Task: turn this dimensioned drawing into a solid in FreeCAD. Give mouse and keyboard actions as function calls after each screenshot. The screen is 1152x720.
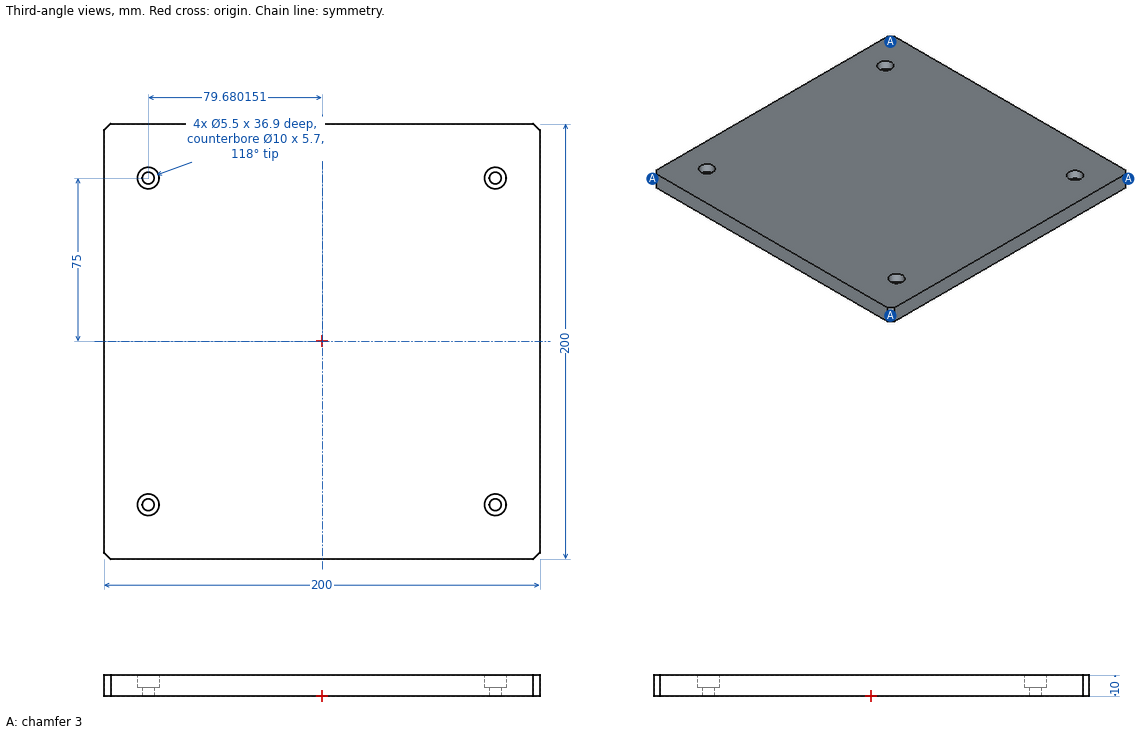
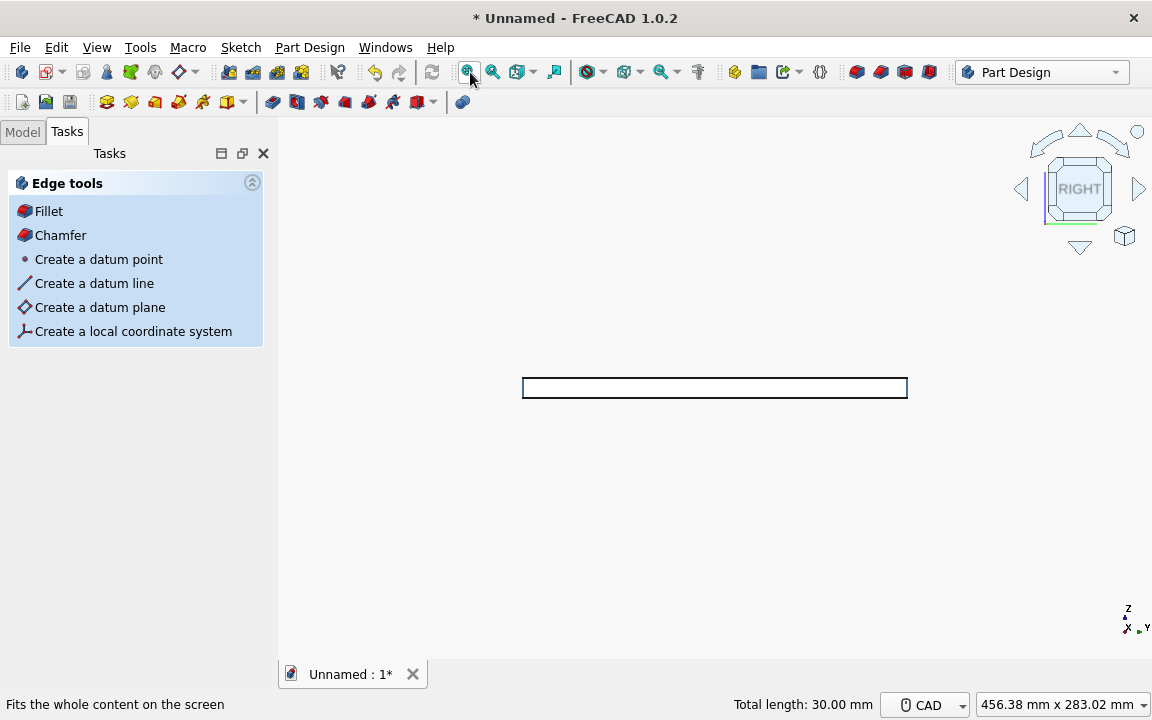
key(5)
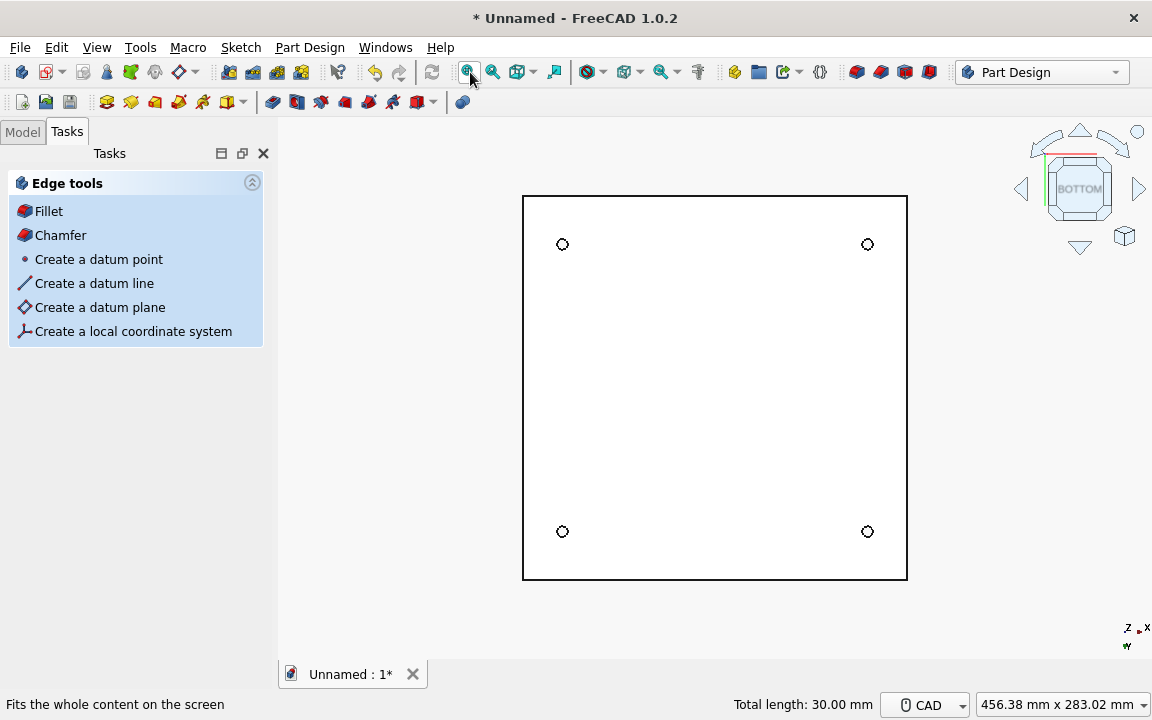
scroll(523, 579, up, 4)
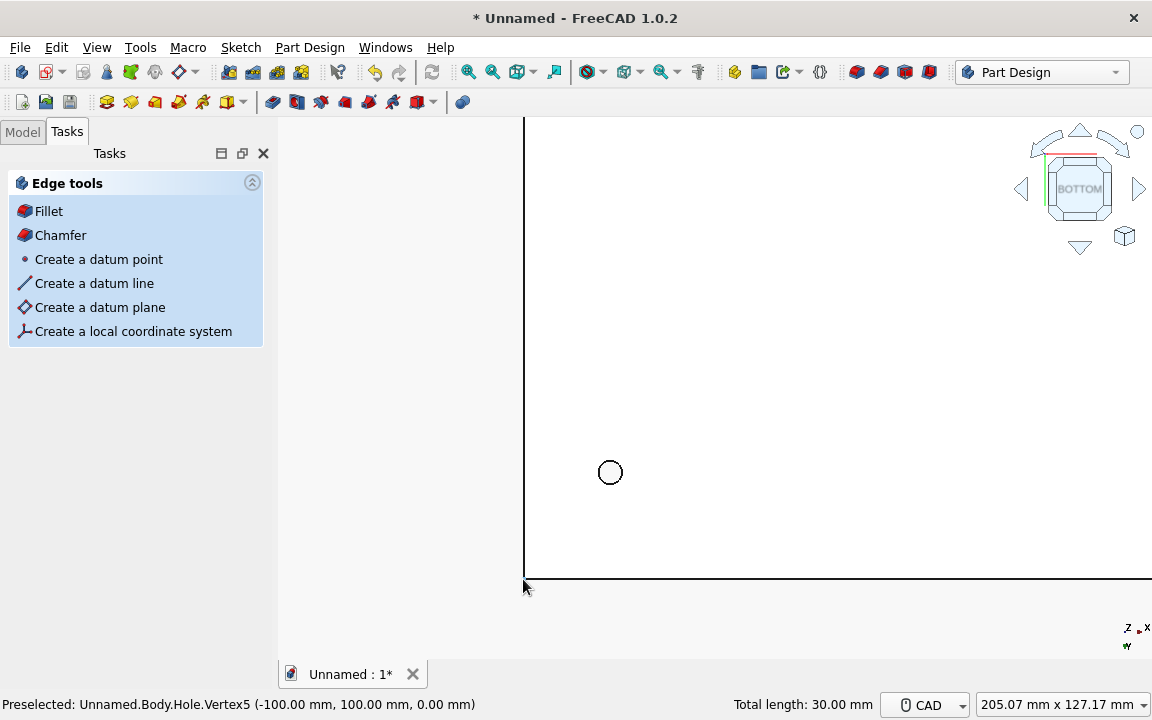
click(470, 72)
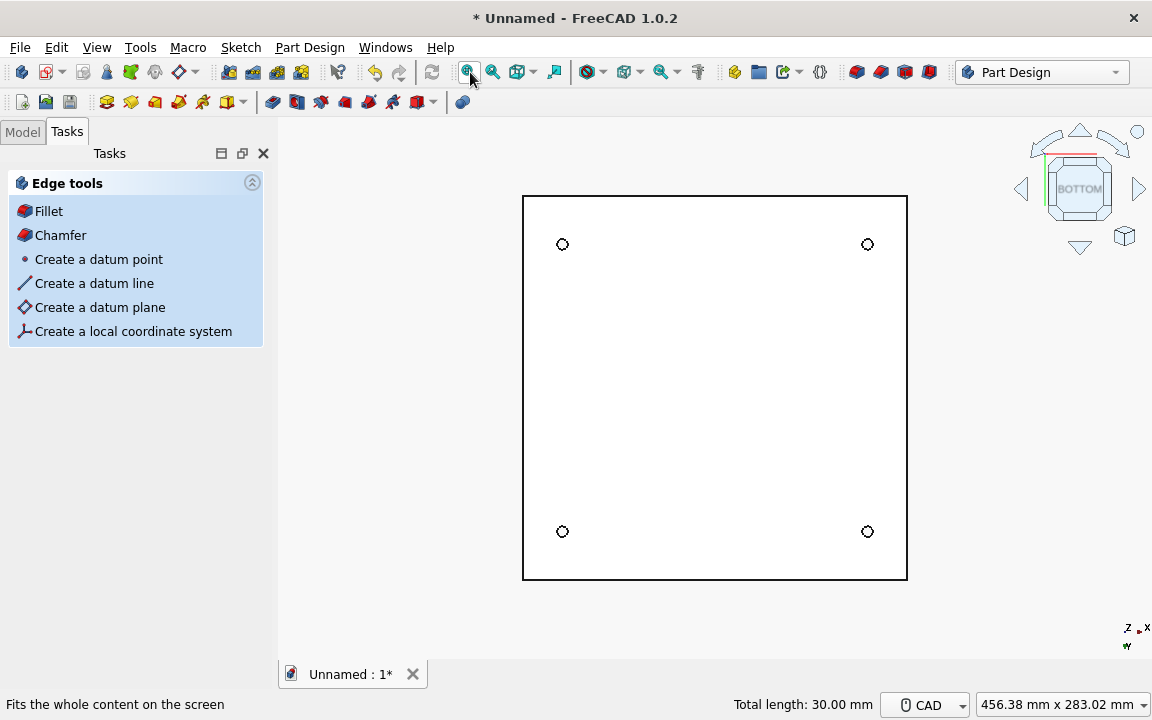
key(4)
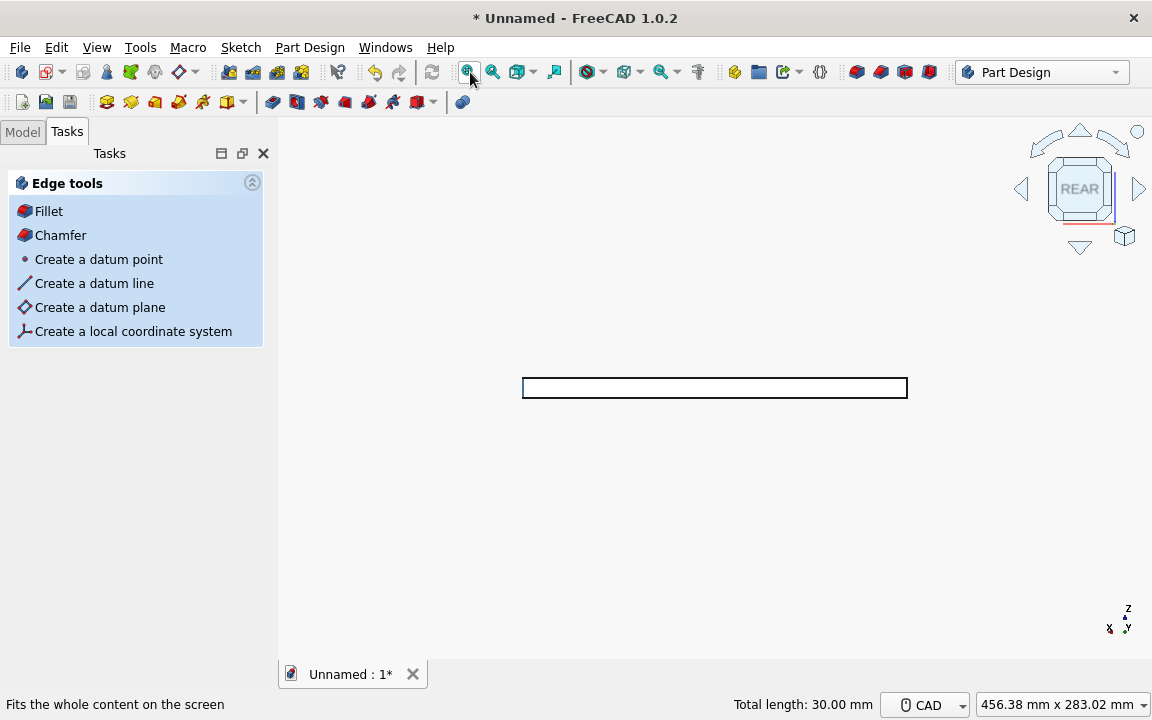
click(470, 72)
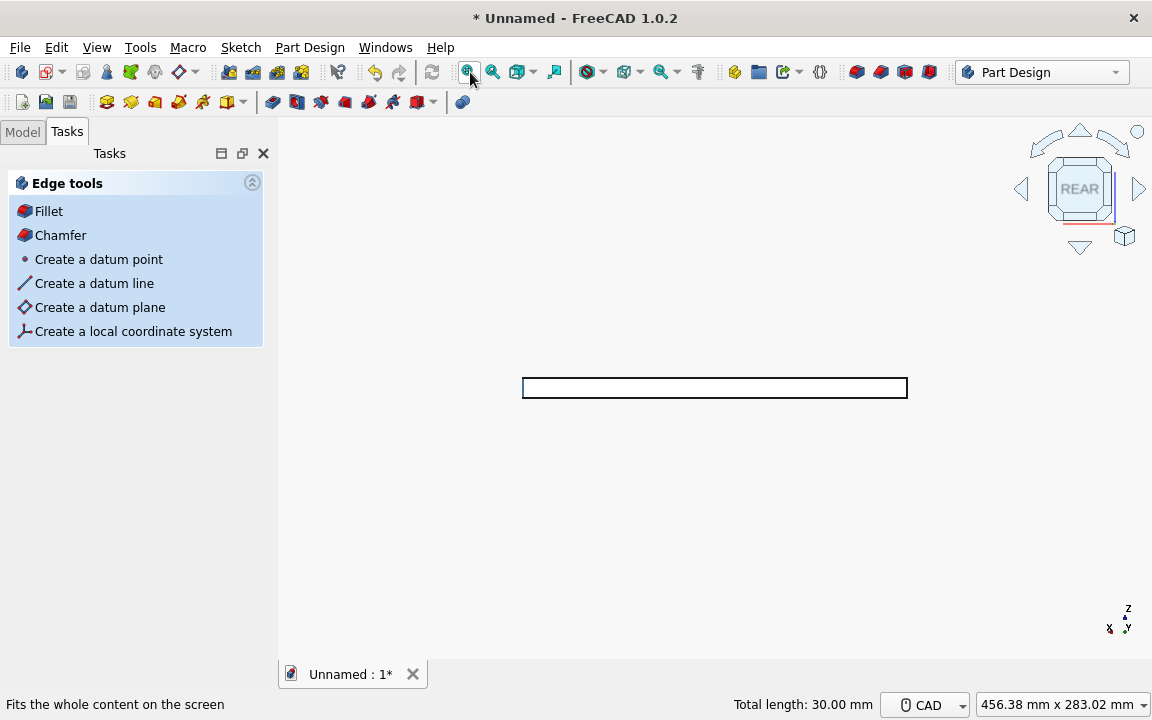
click(907, 387, ctrl)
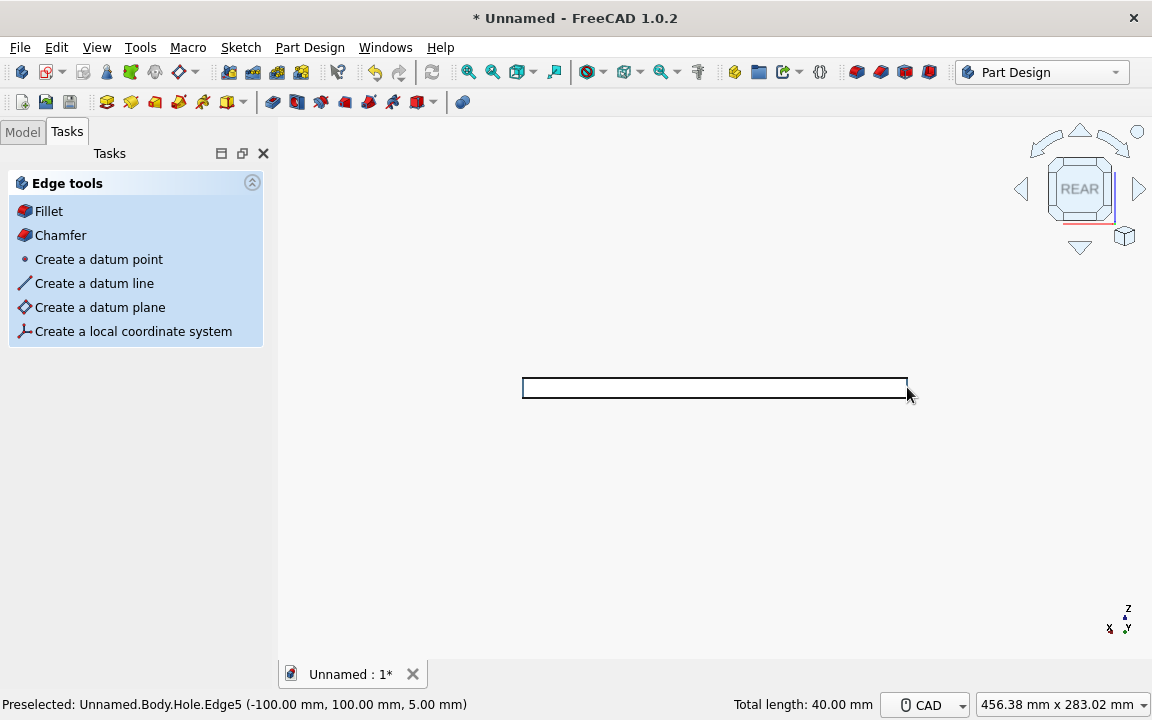
click(882, 72)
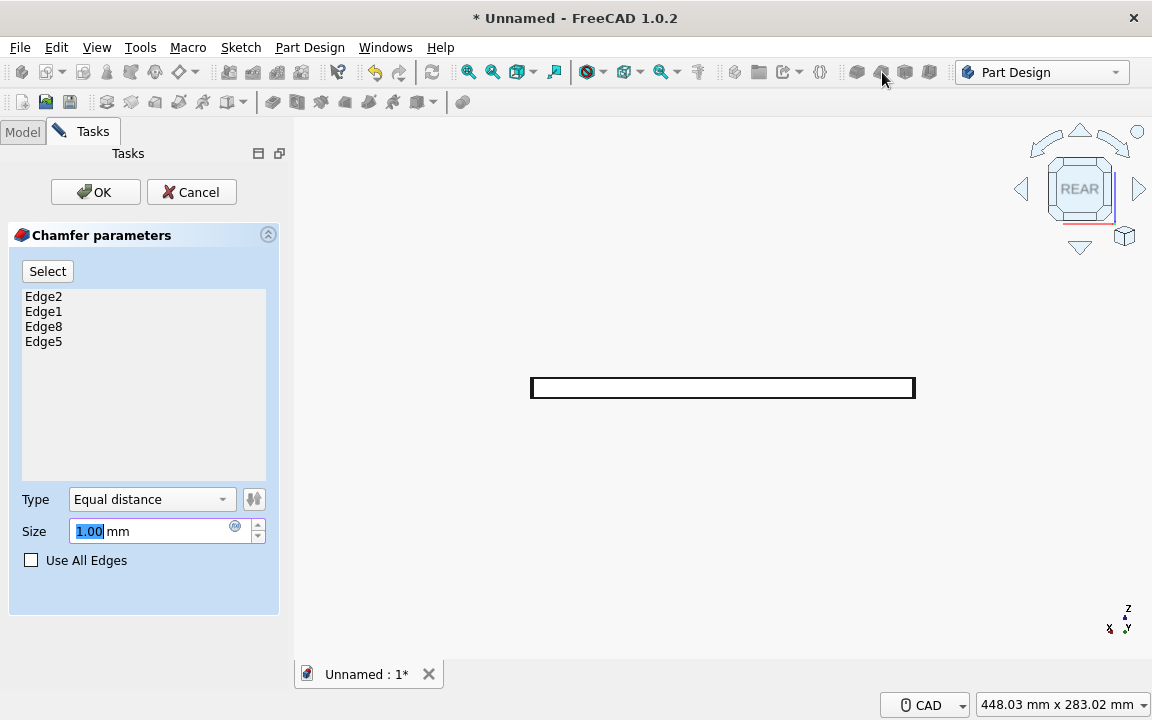
text(3)
key(Tab)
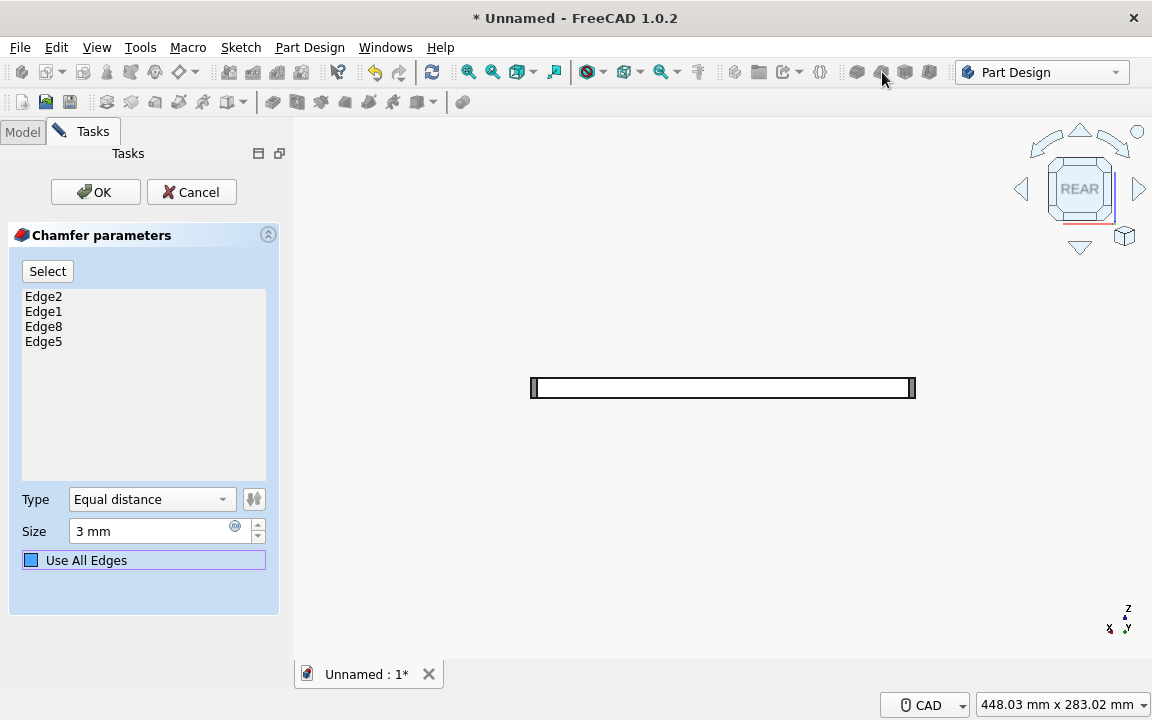
click(96, 192)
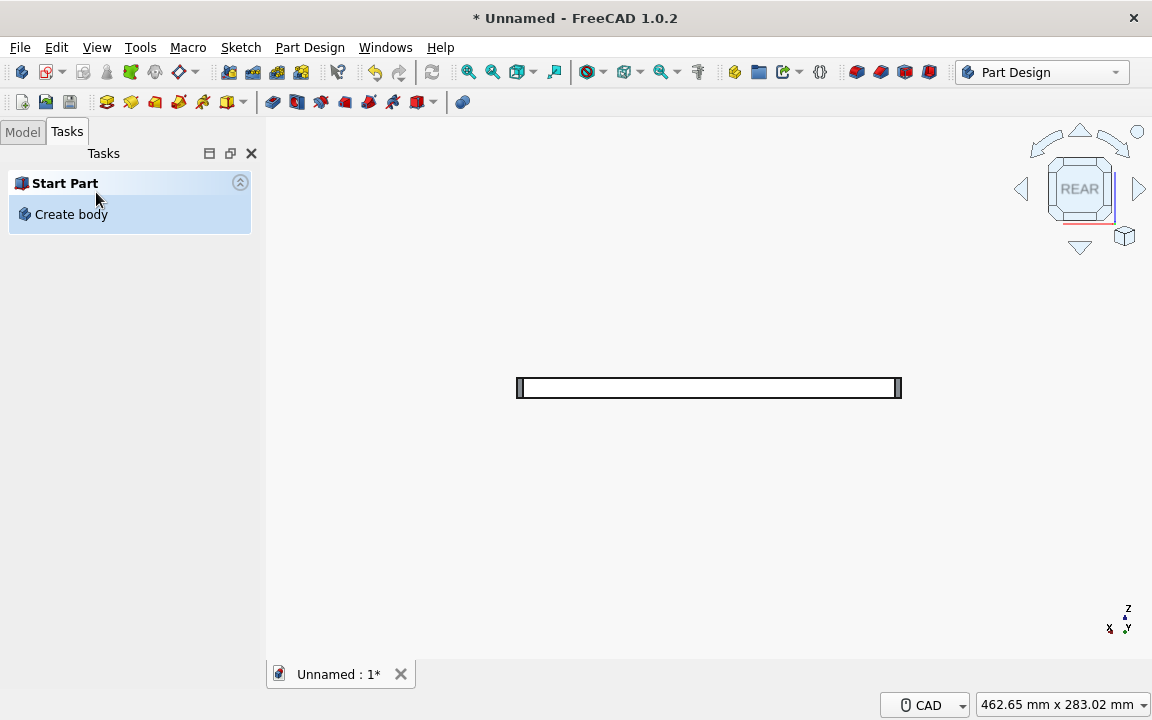
key(0)